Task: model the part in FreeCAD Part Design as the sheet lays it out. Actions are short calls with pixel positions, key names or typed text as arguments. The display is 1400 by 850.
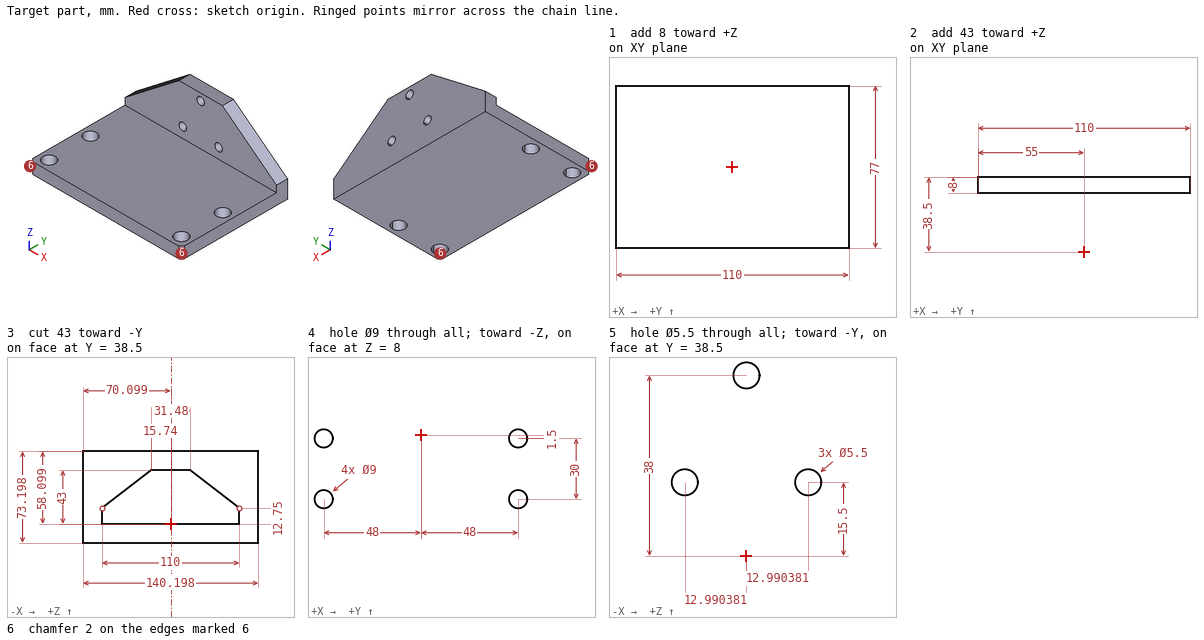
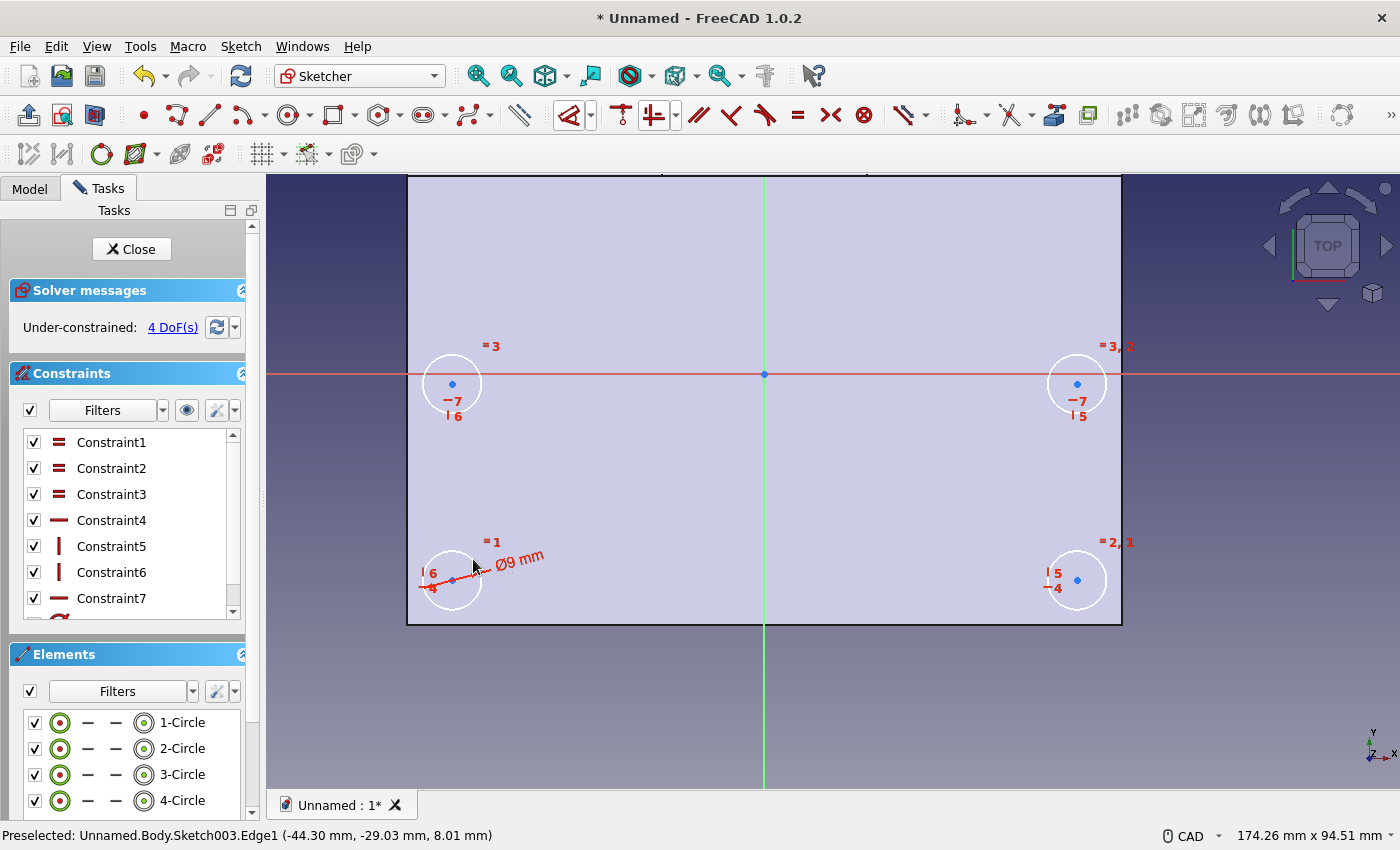
click(452, 580)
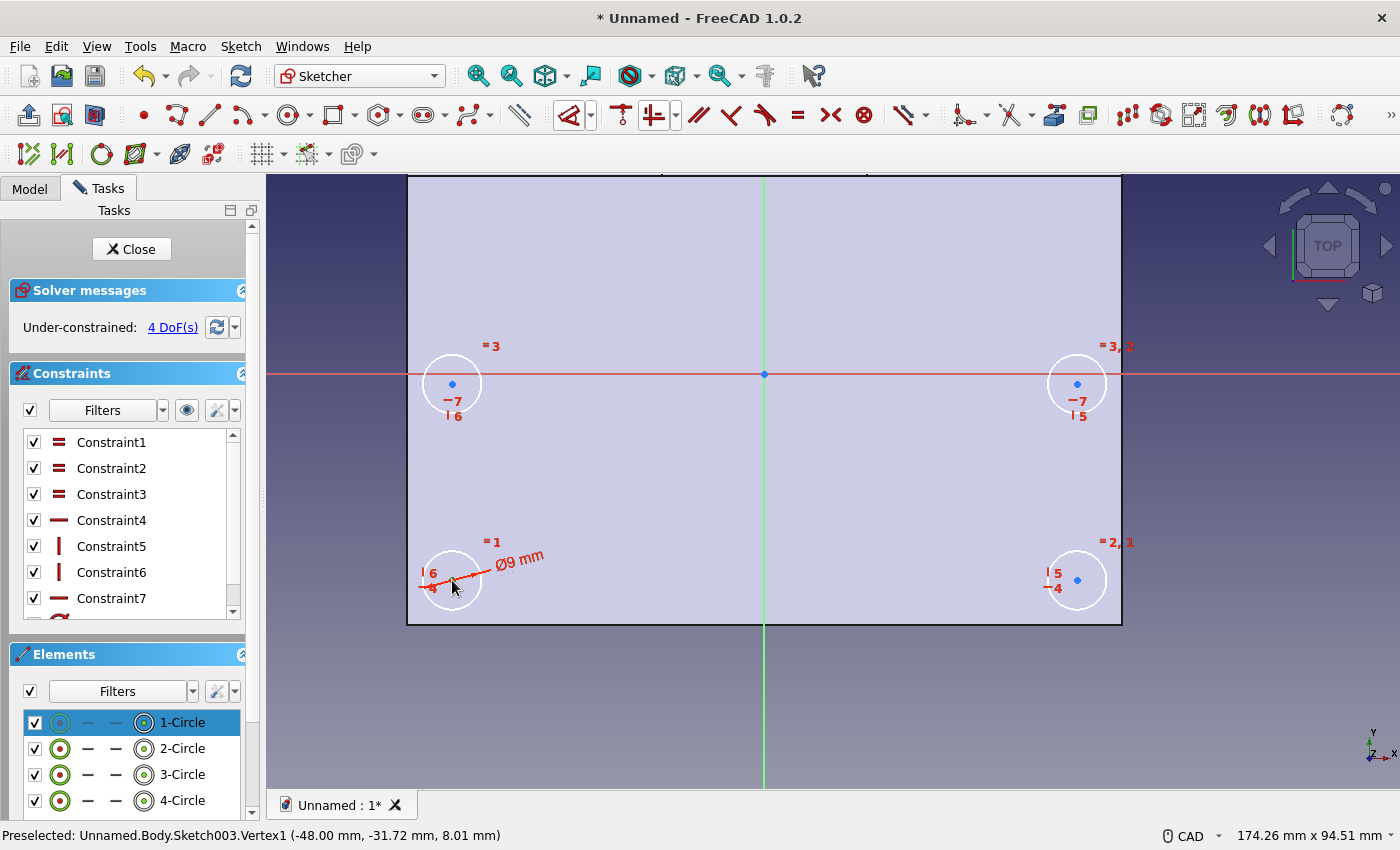
key(l)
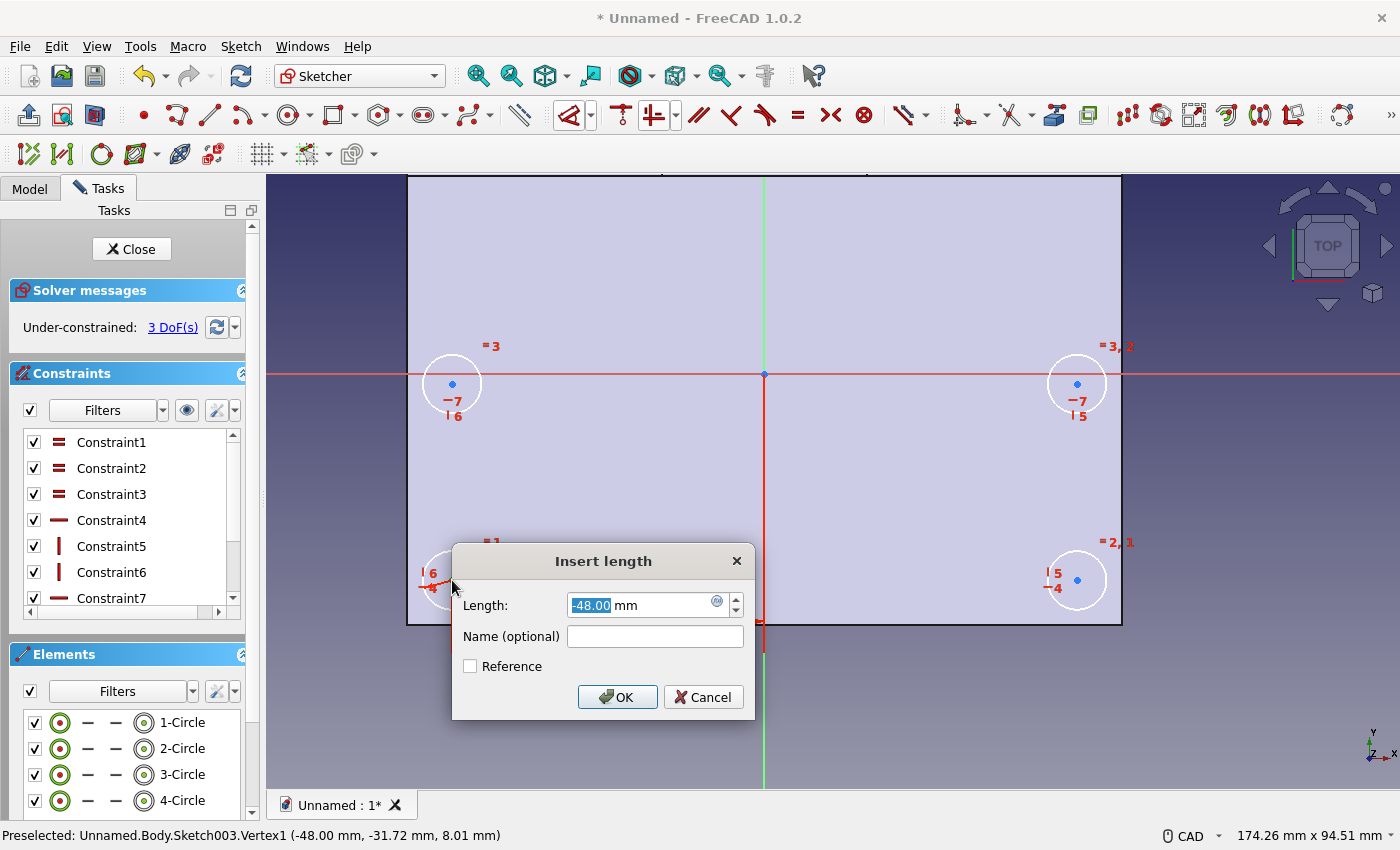
text(-48)
key(Return)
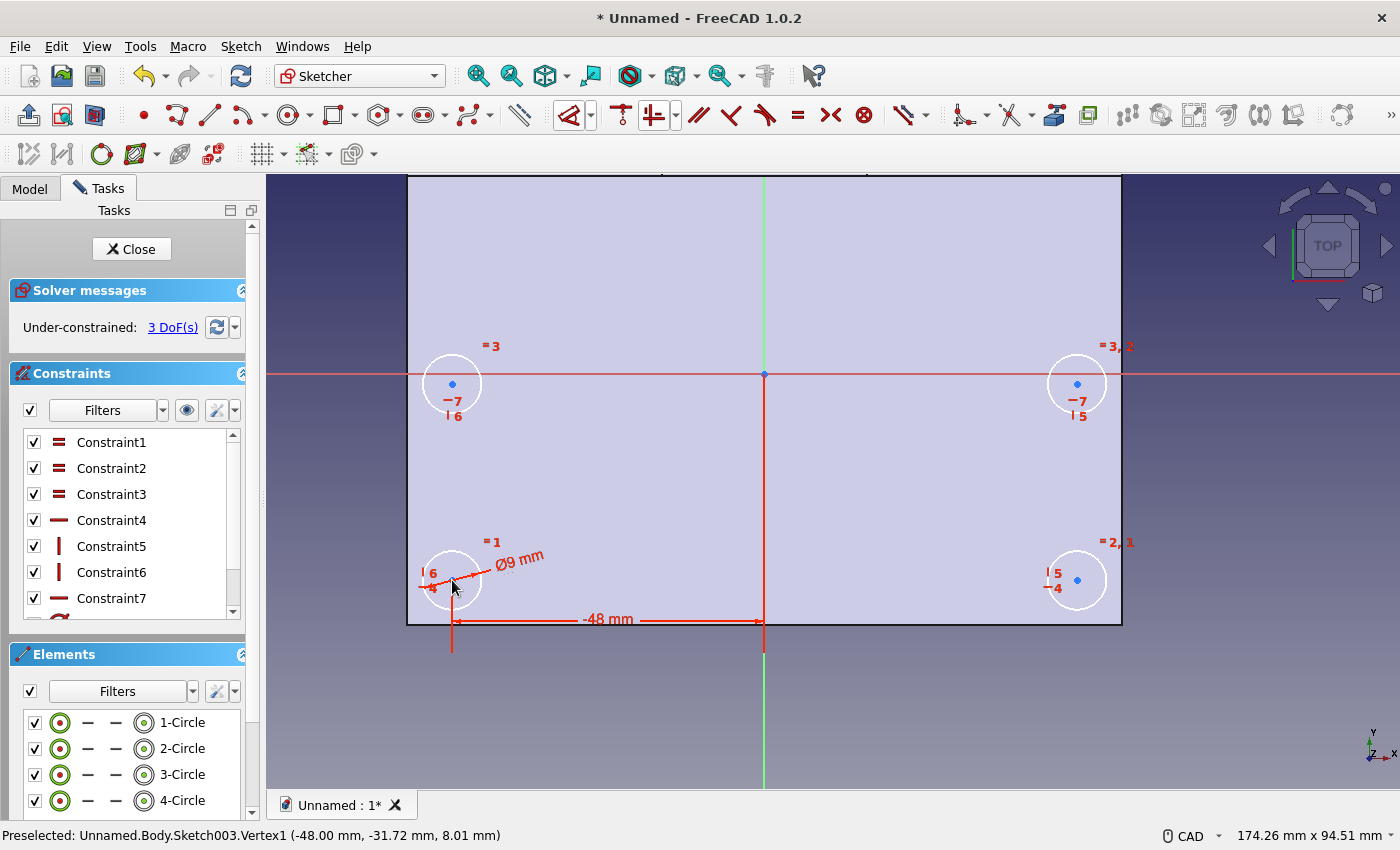
click(1077, 580)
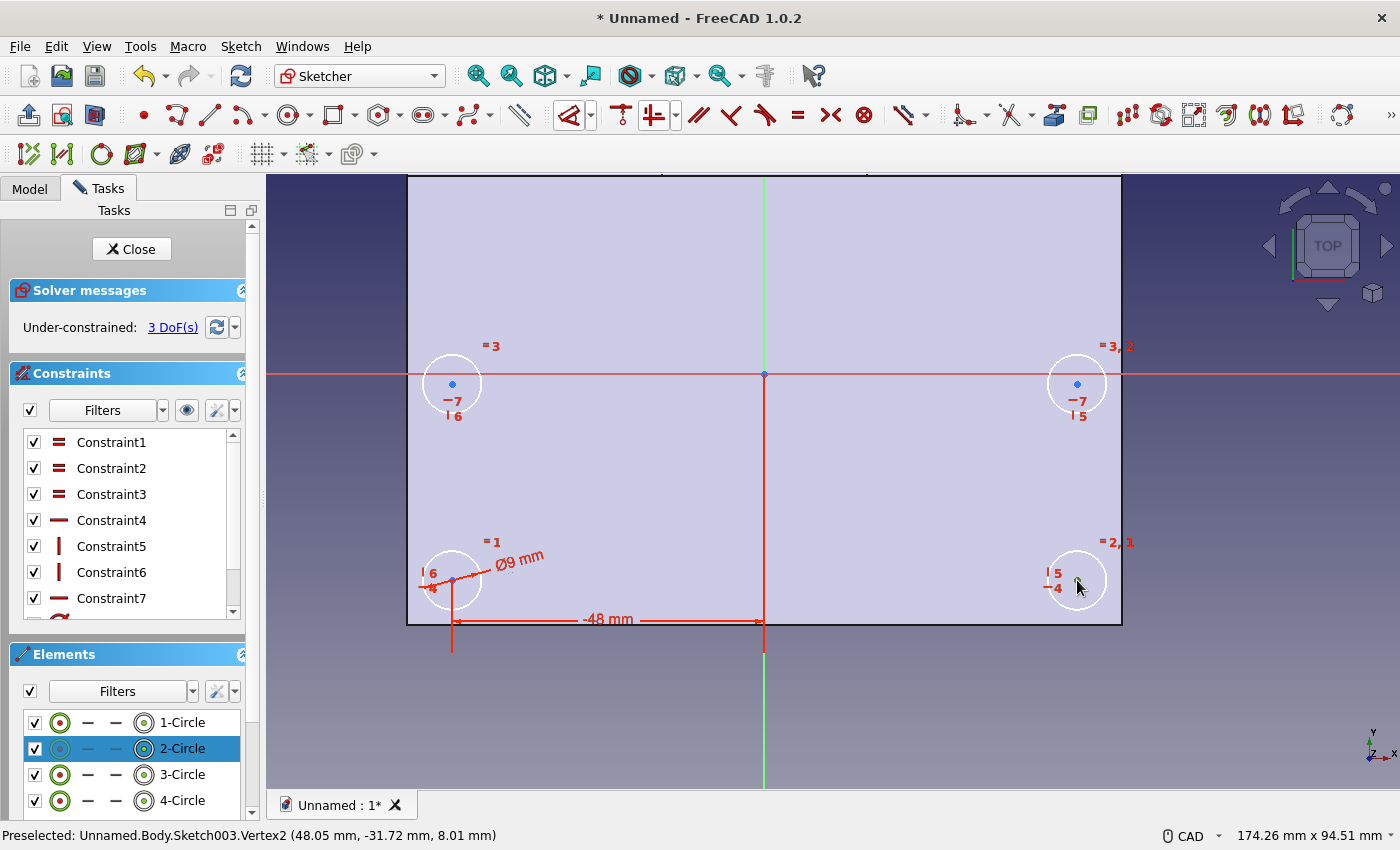
click(590, 116)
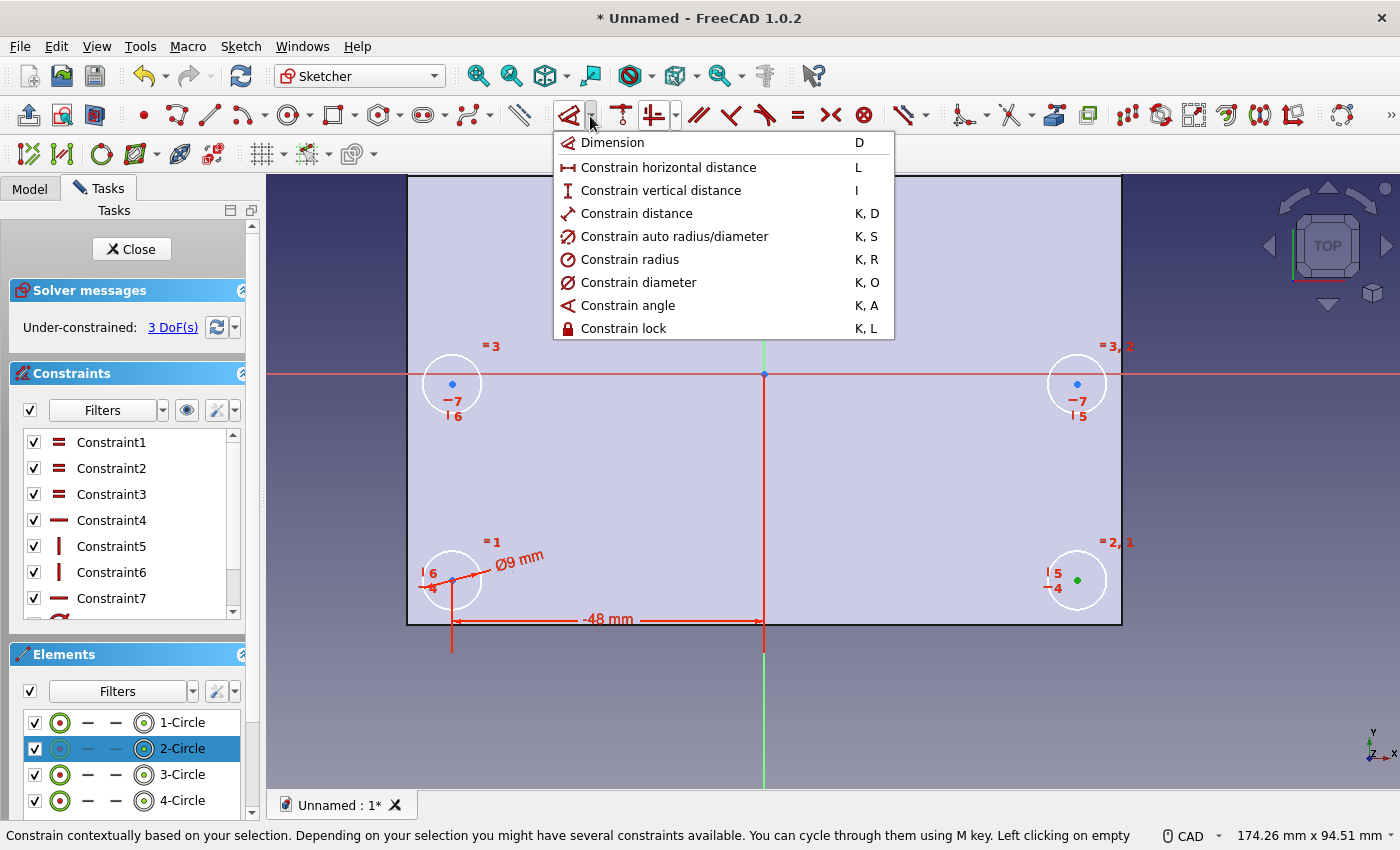
click(724, 168)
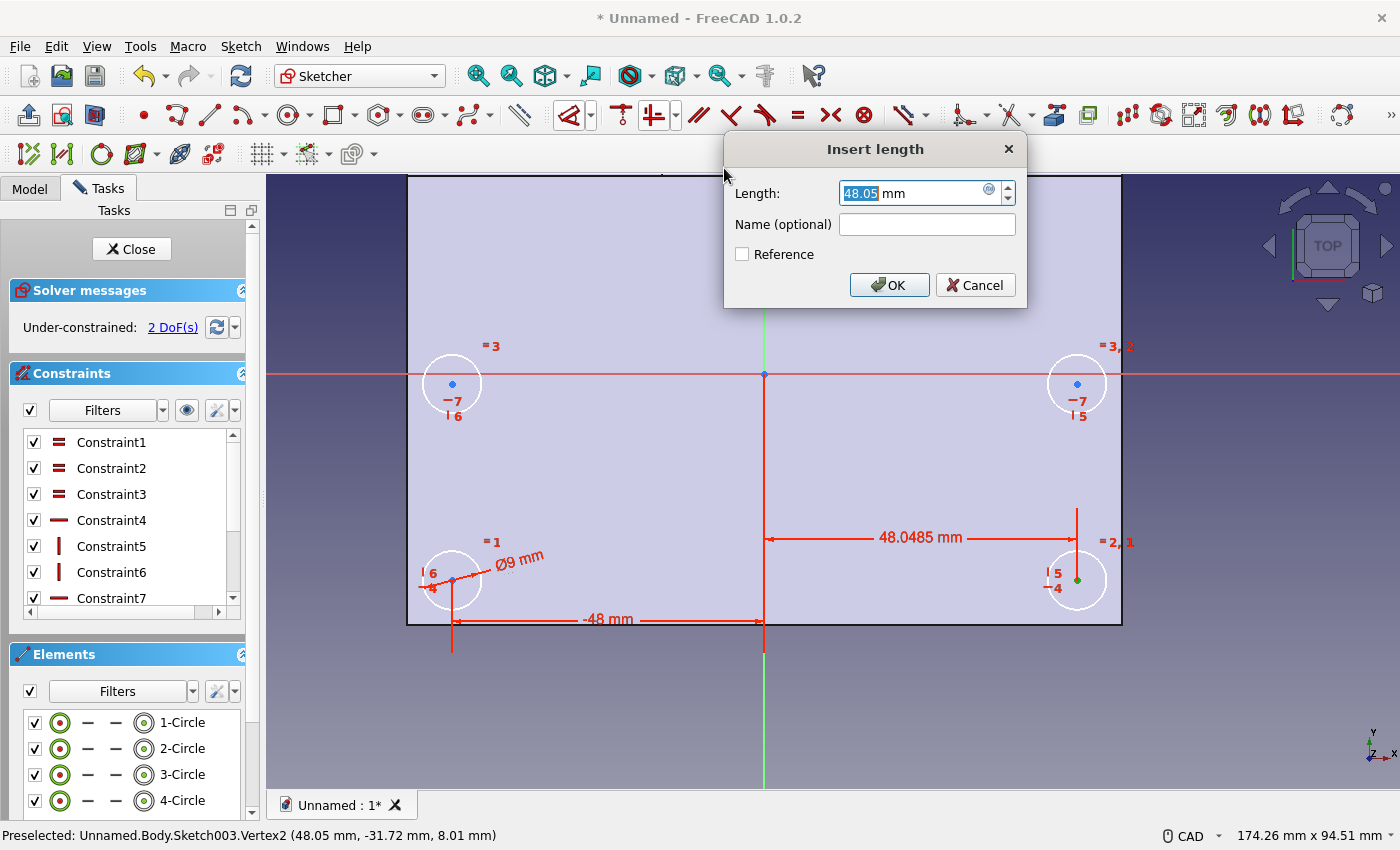
text(48)
key(Return)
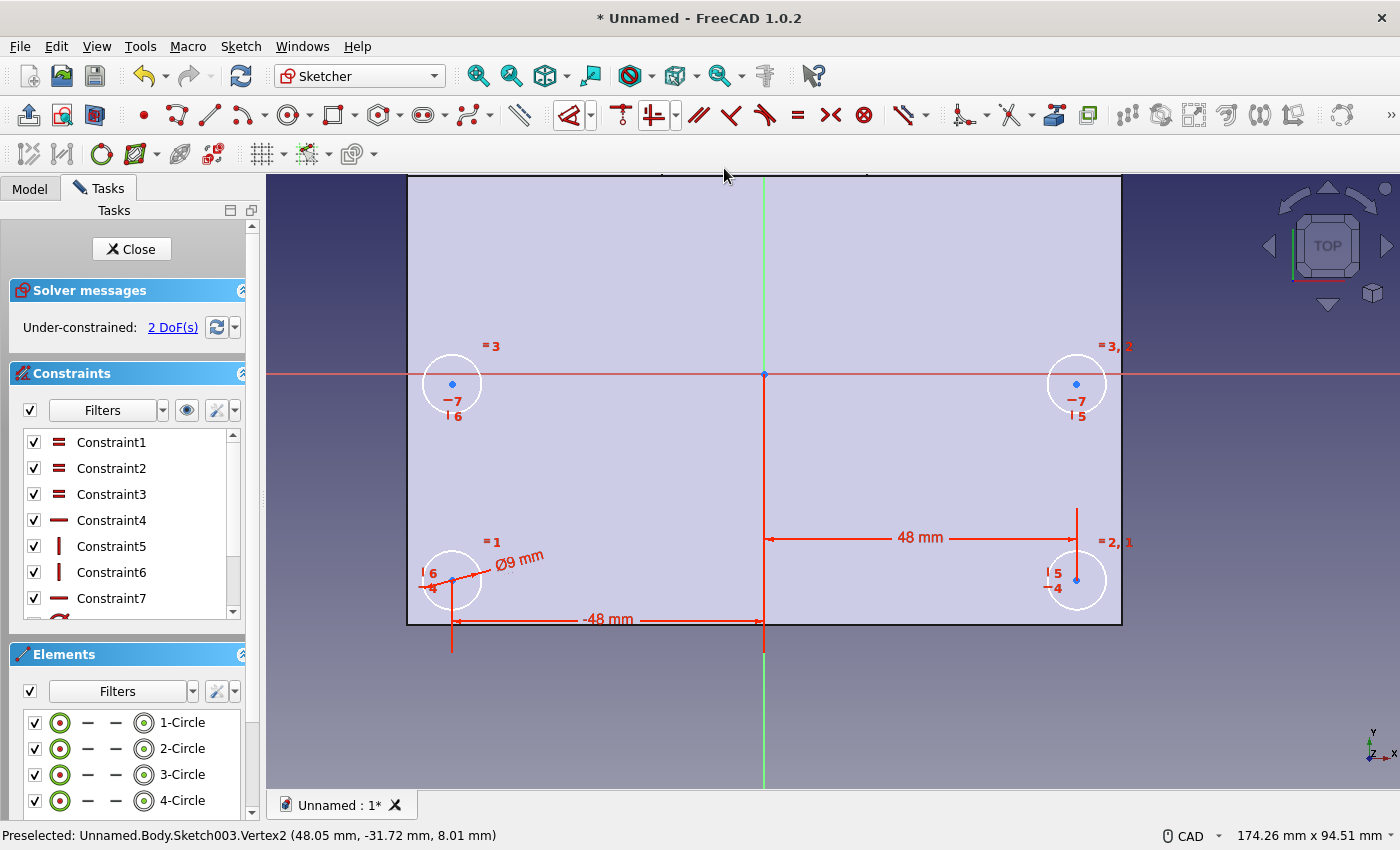
scroll(1077, 384, up, 8)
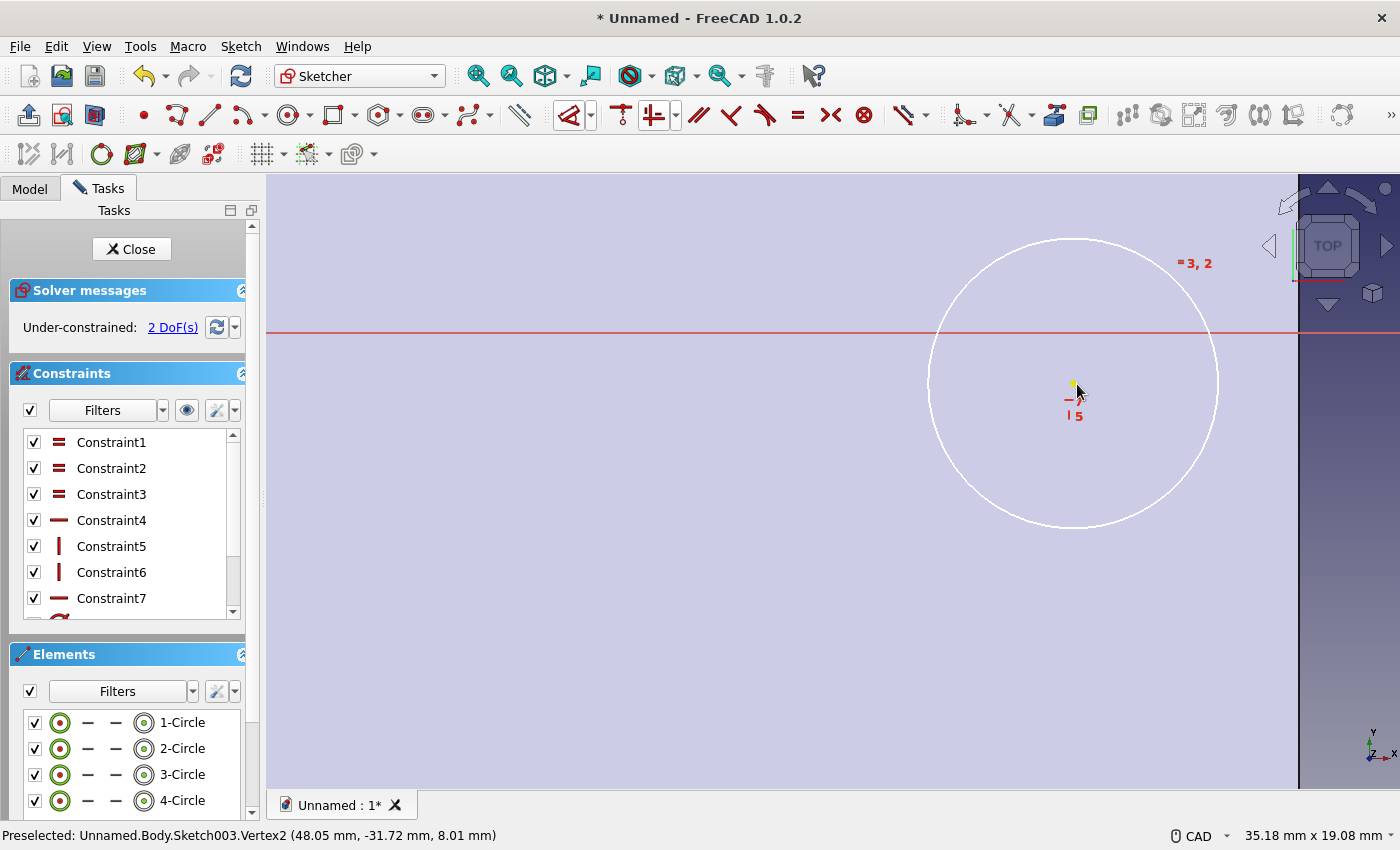
click(1073, 383)